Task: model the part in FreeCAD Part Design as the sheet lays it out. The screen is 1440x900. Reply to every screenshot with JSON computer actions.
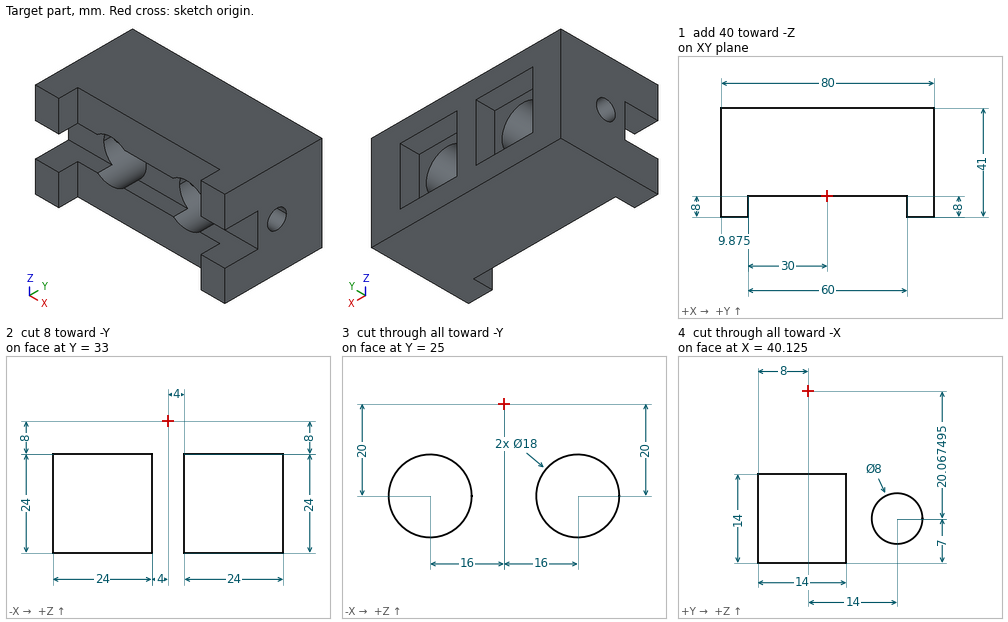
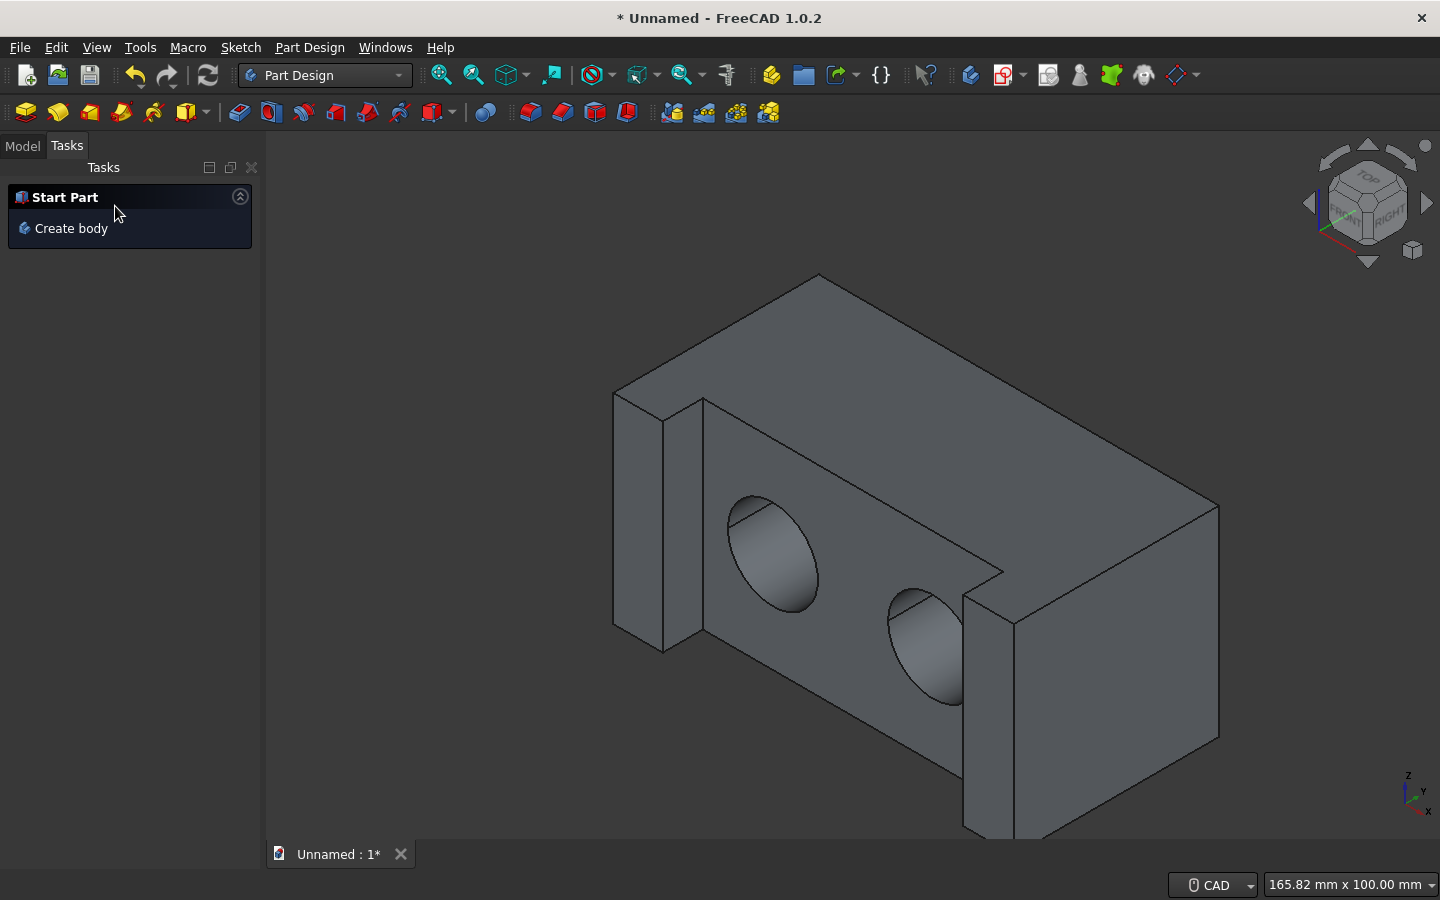
{"action": "left_click", "coordinate": [442, 76]}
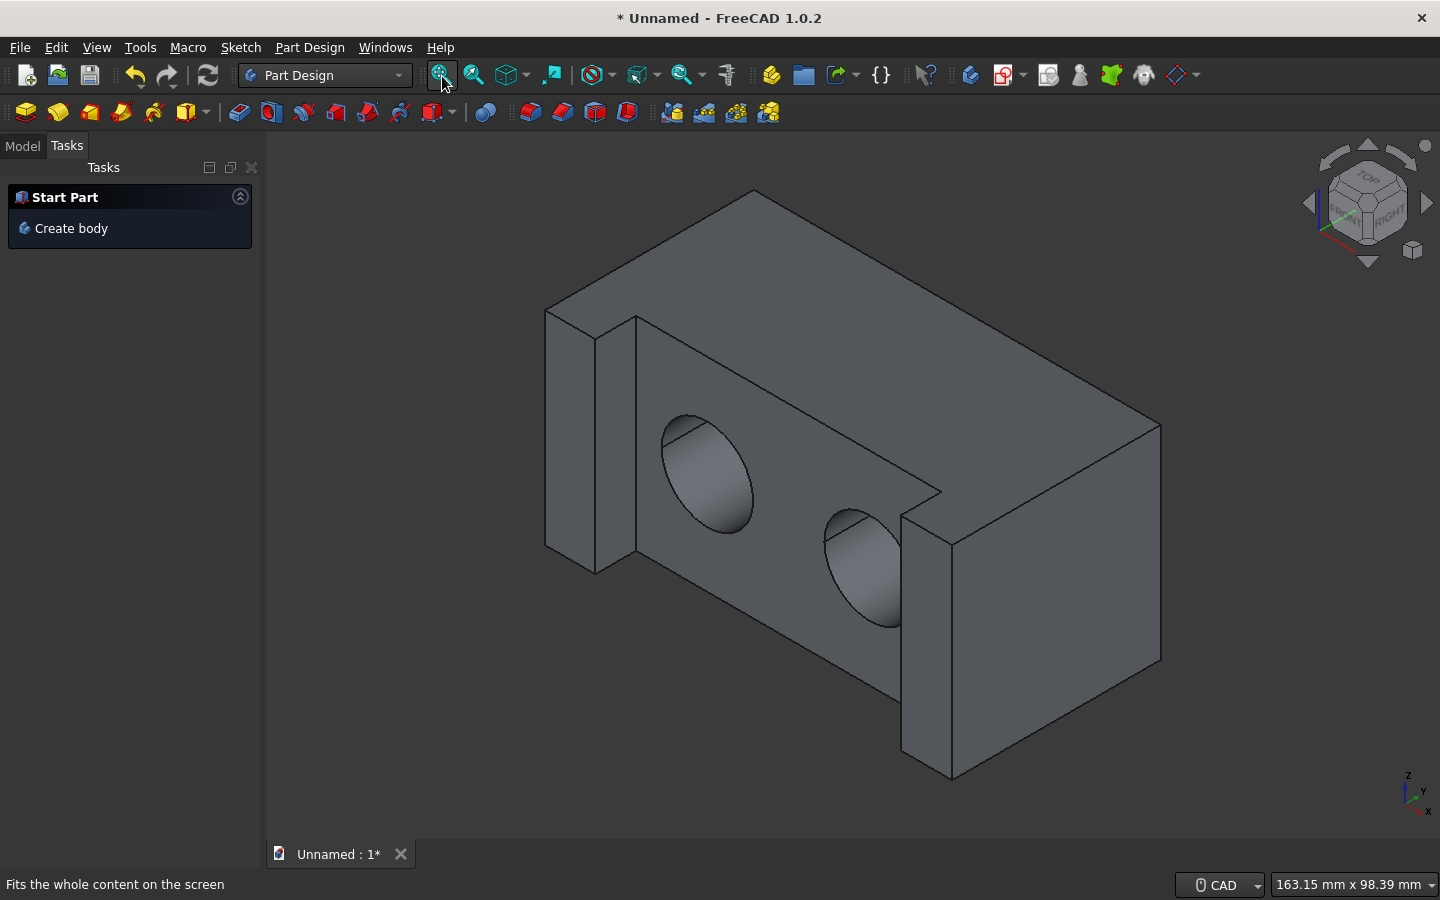
{"action": "left_click", "coordinate": [1057, 602]}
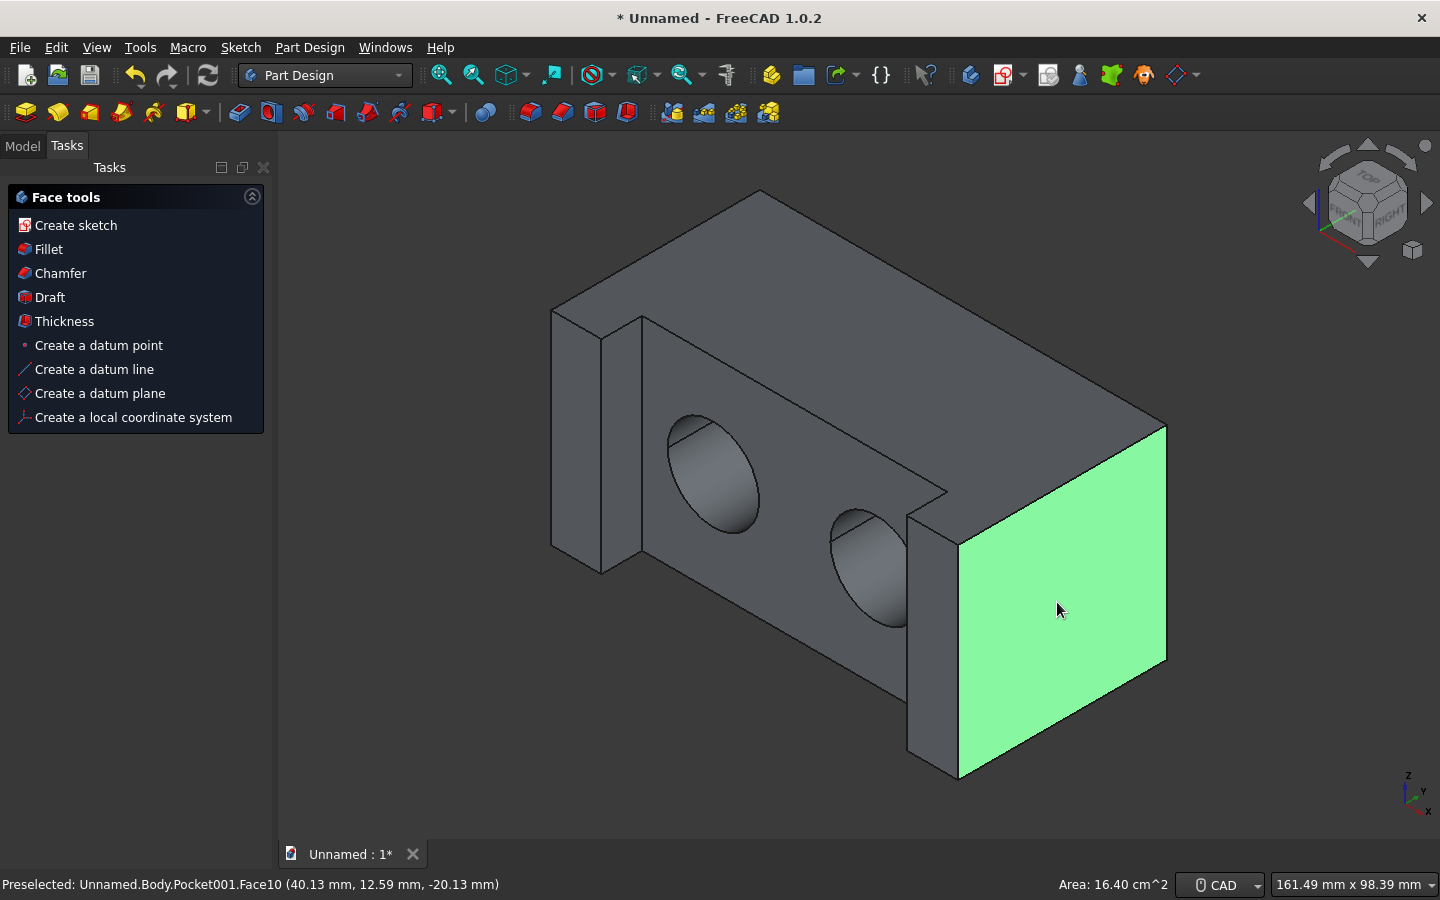
{"action": "left_click", "coordinate": [1004, 76]}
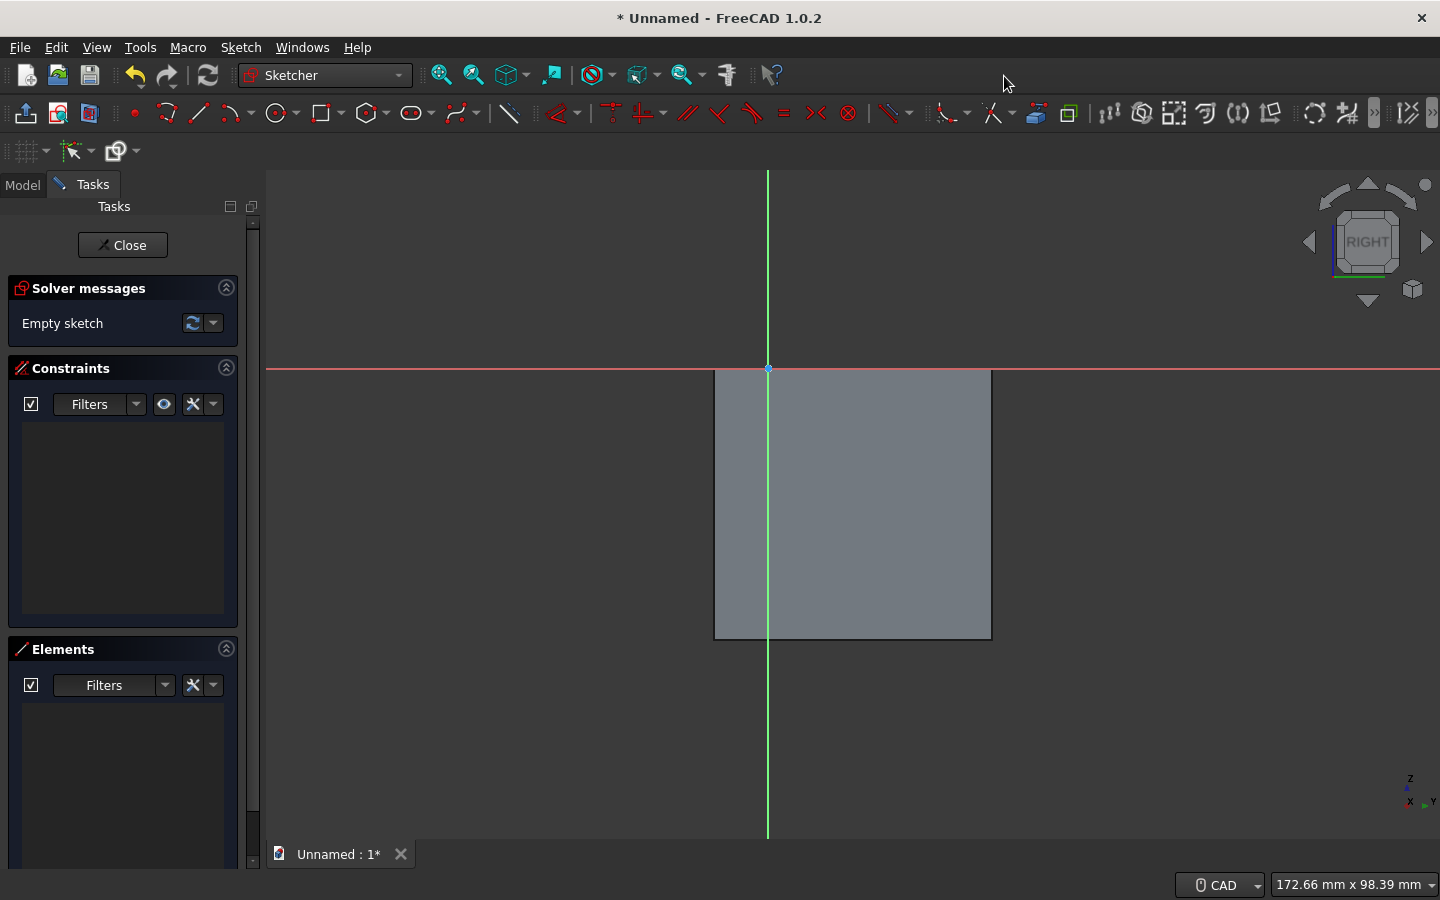
{"action": "scroll", "coordinate": [816, 425], "scroll_direction": "up", "scroll_amount": 4}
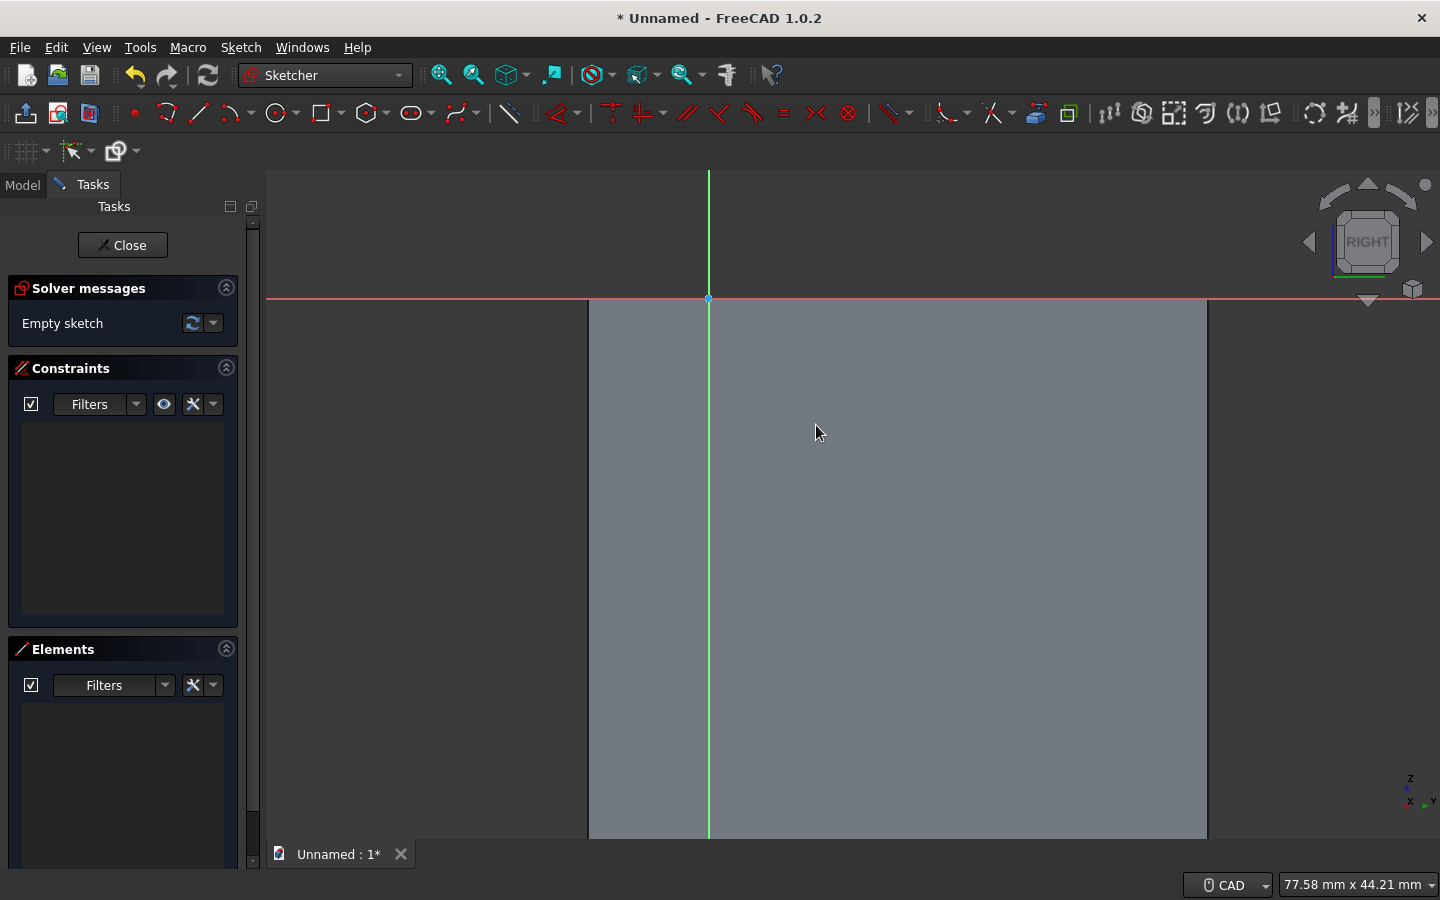
{"action": "left_click", "coordinate": [322, 114]}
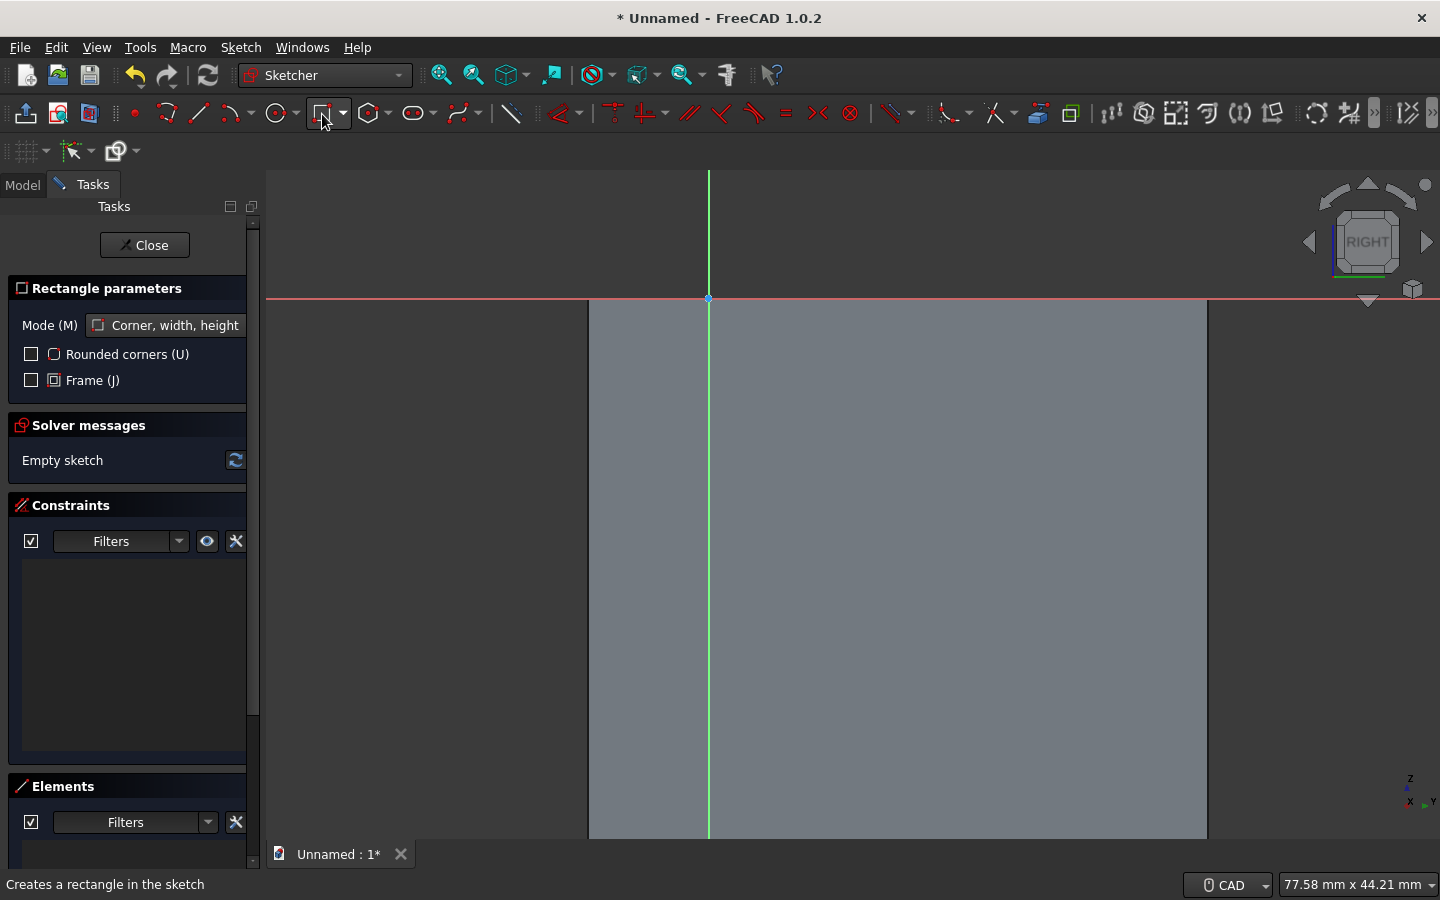
{"action": "left_click", "coordinate": [588, 497]}
{"action": "left_click", "coordinate": [799, 708]}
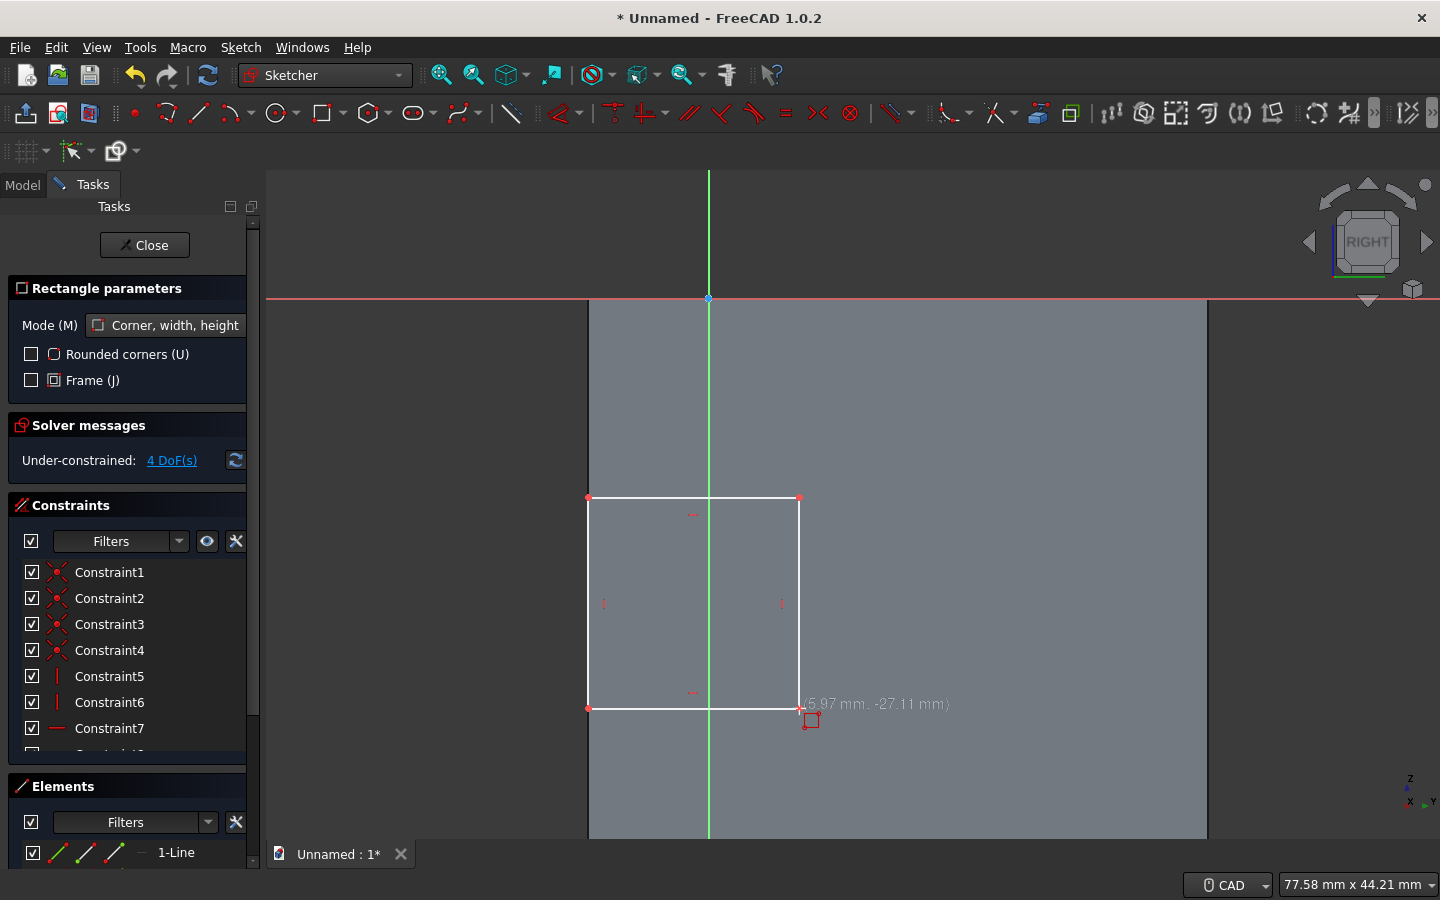
{"action": "left_click", "coordinate": [276, 114]}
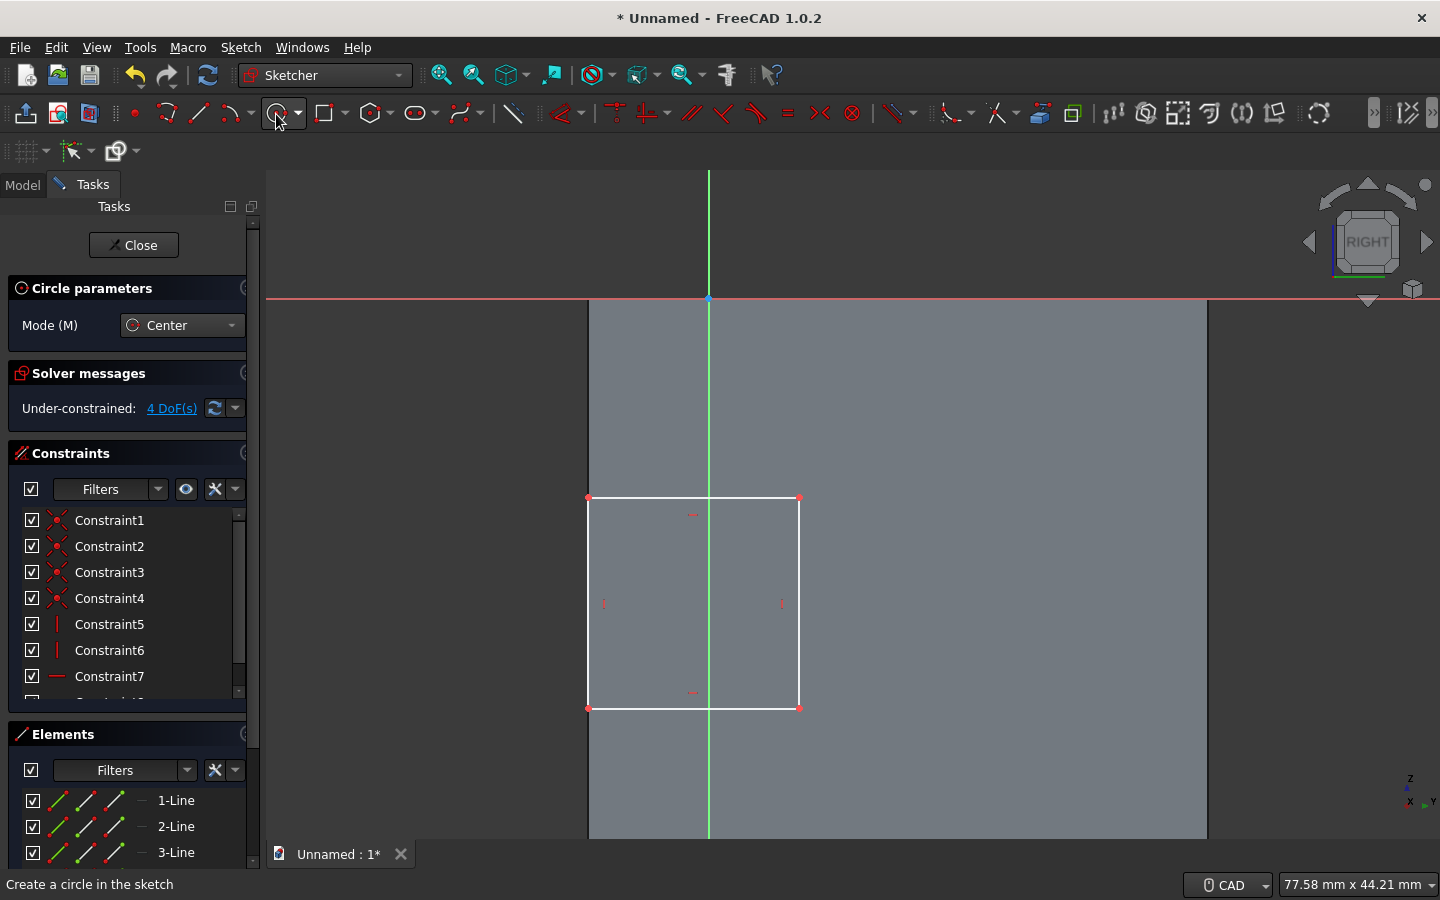
{"action": "left_click", "coordinate": [920, 602]}
{"action": "left_click", "coordinate": [963, 560]}
{"action": "key", "text": "Escape"}